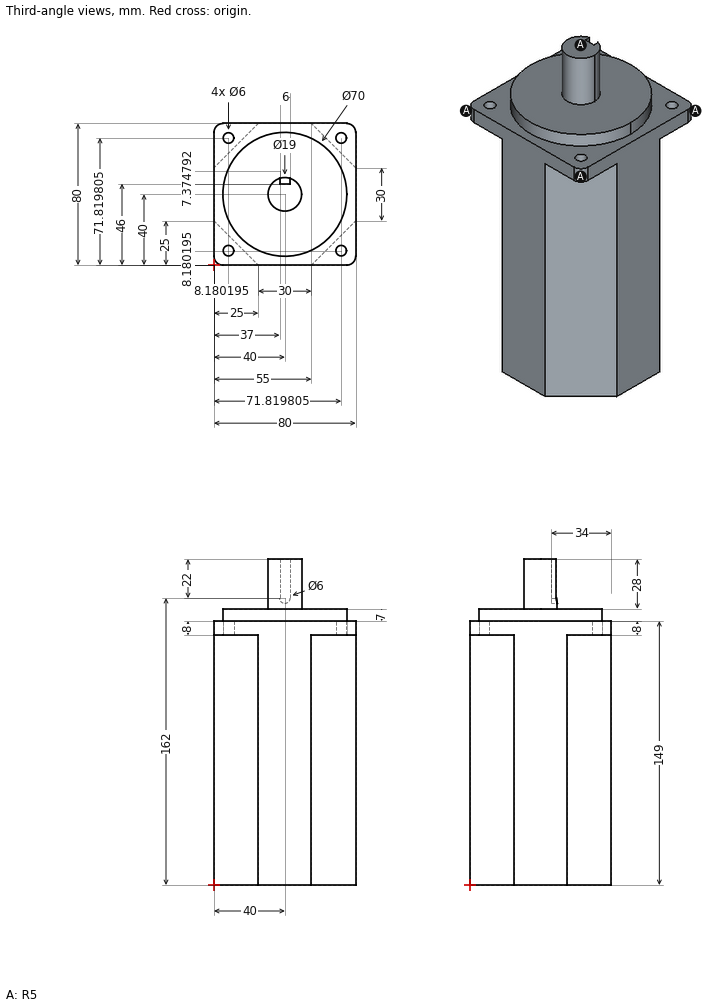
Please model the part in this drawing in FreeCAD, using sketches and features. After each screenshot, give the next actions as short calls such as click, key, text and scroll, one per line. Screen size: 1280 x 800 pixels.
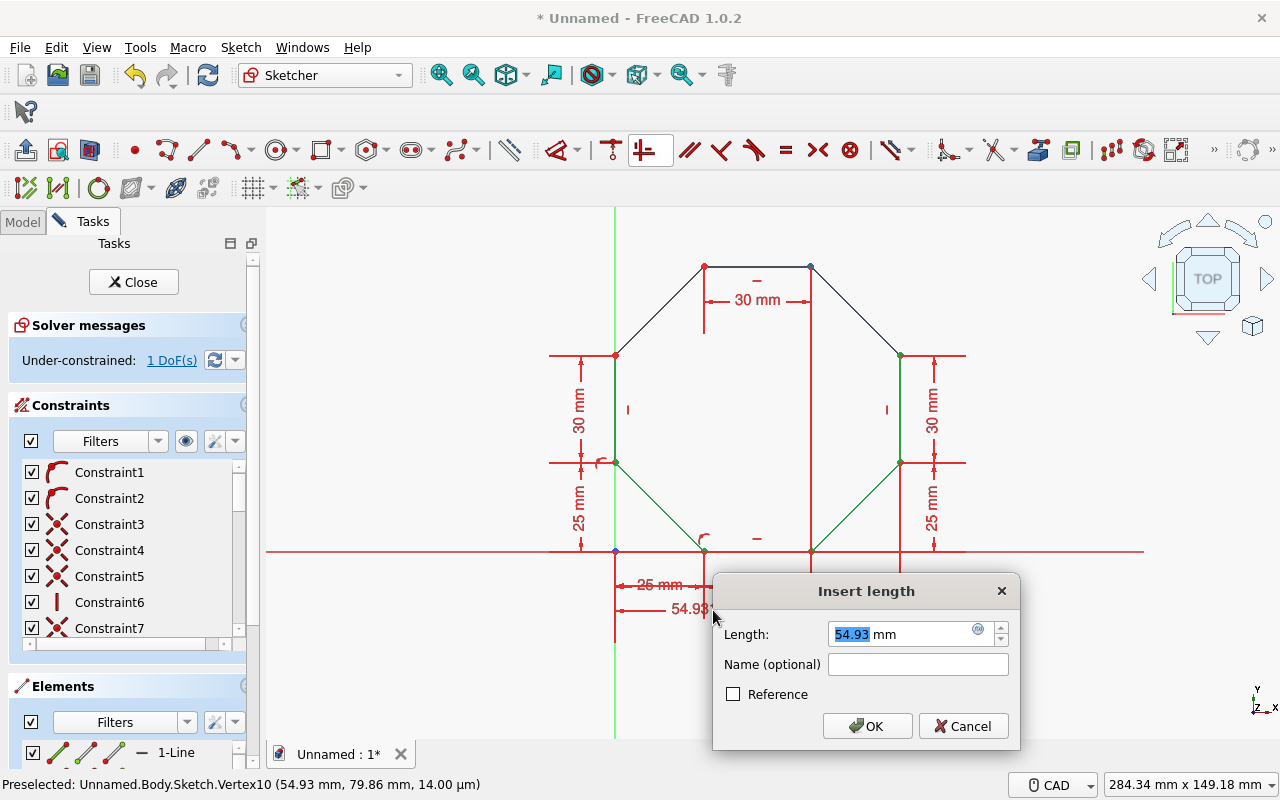
text(55)
key(Return)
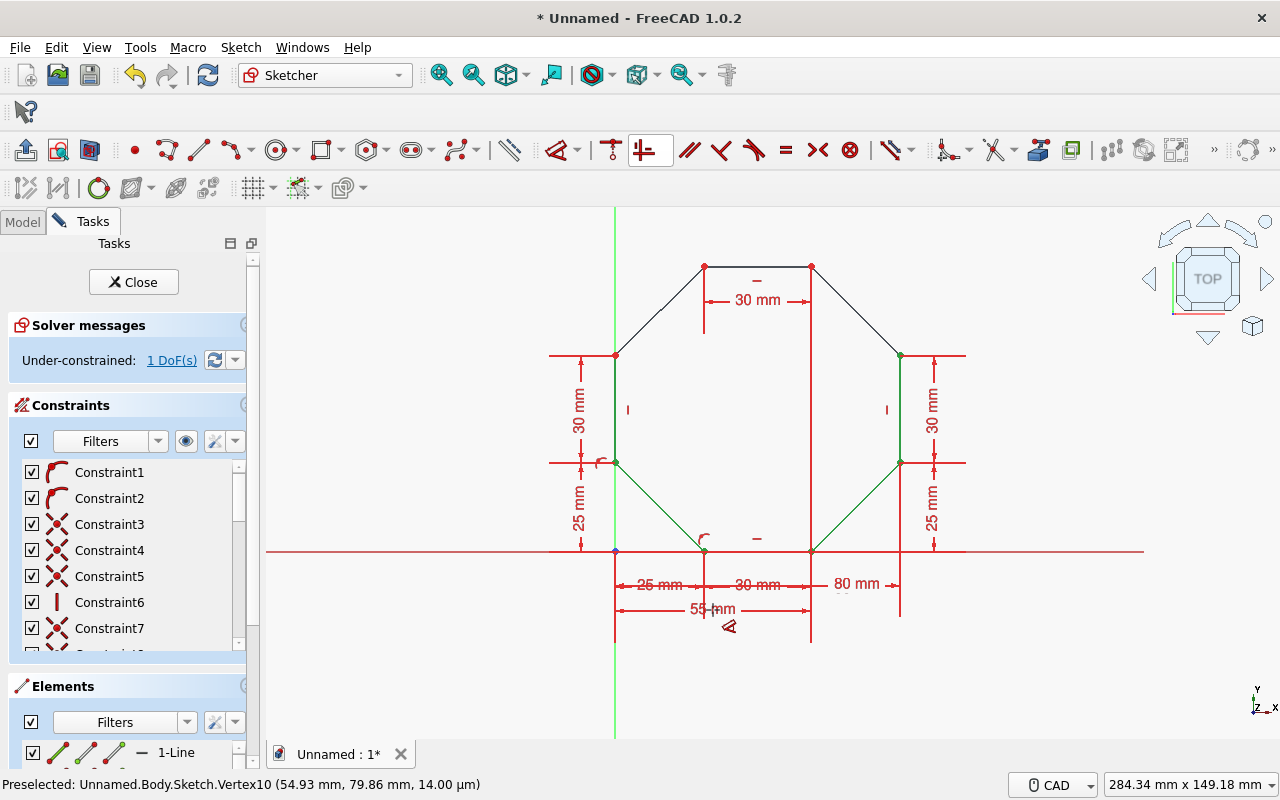
click(811, 267)
click(581, 344)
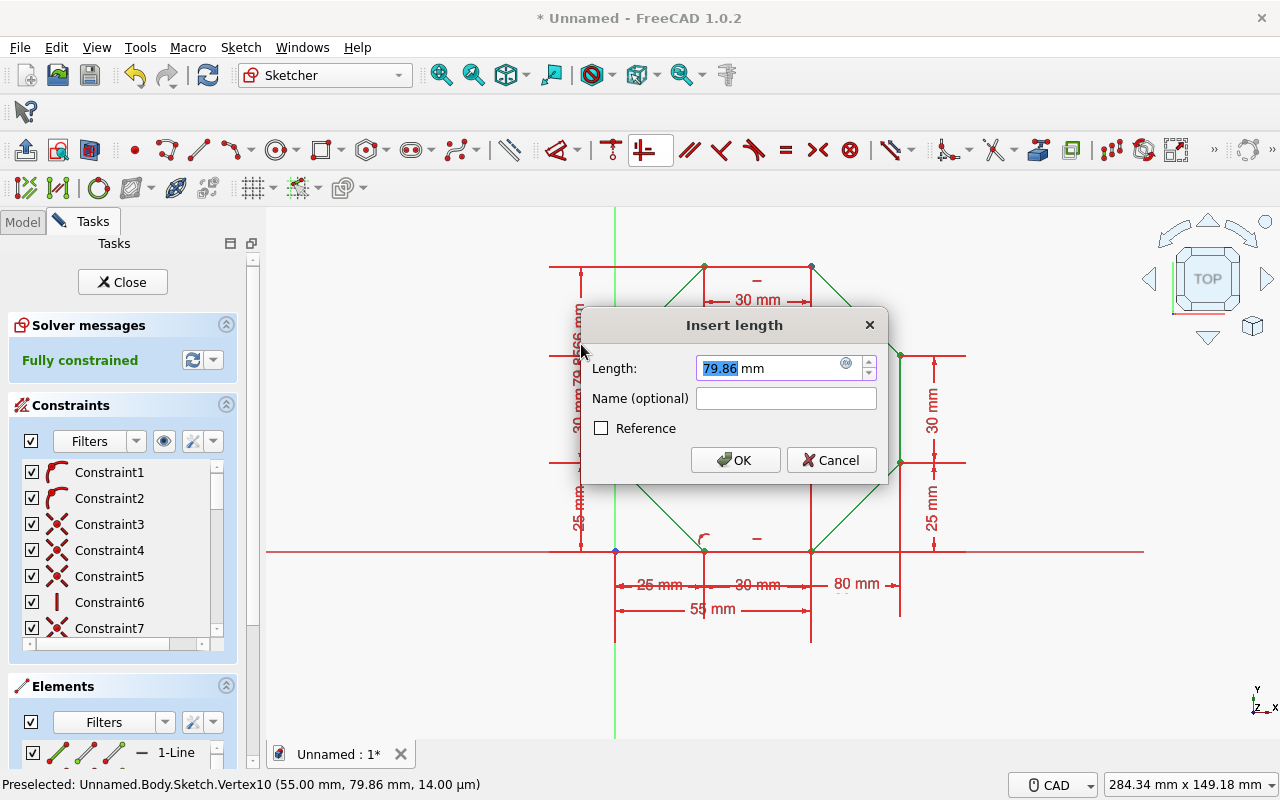
text(80)
key(Return)
key(Escape)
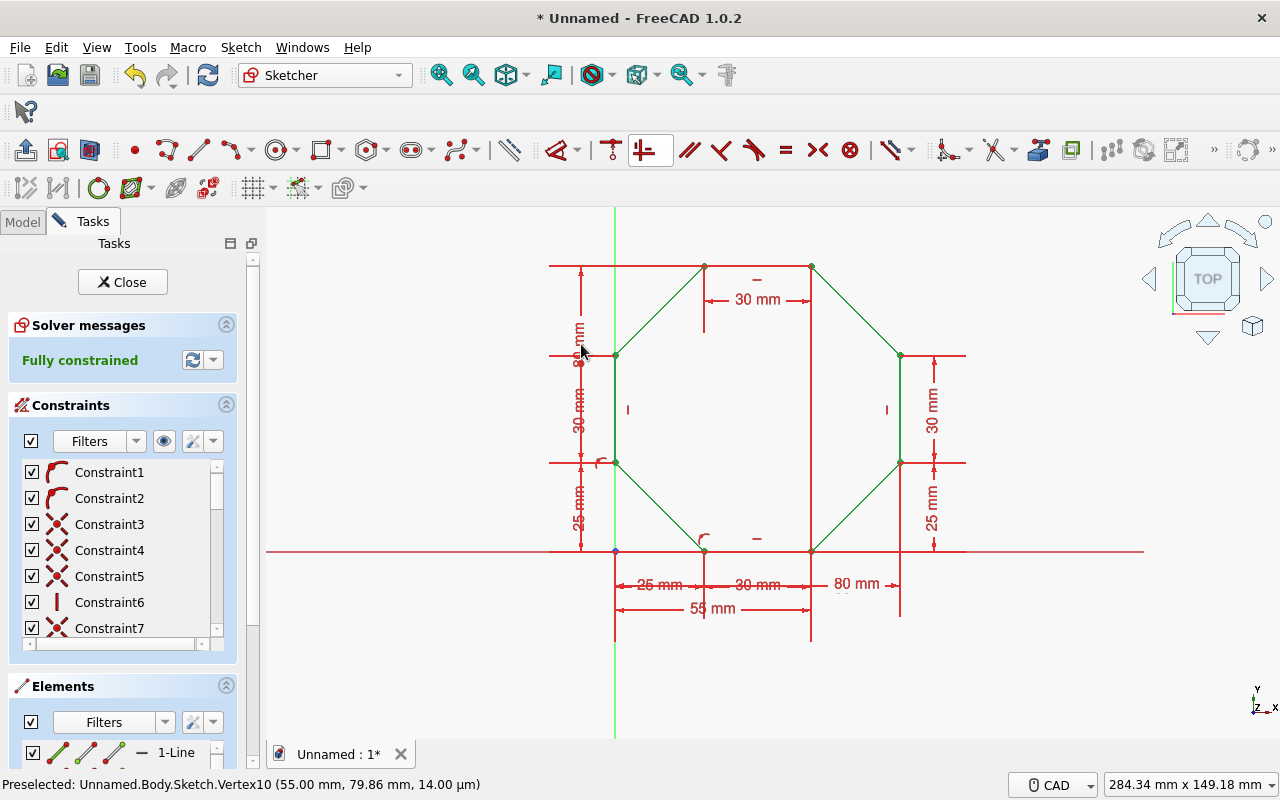
click(123, 282)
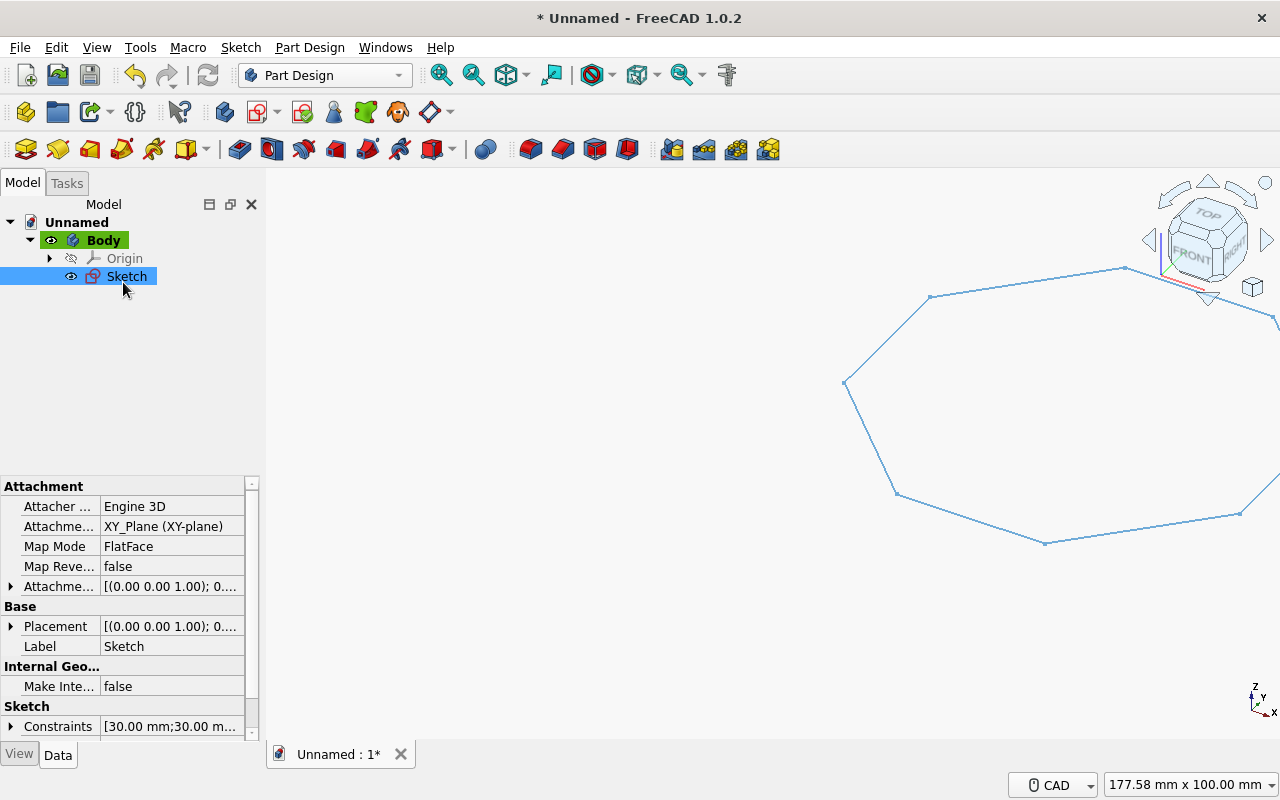
click(26, 150)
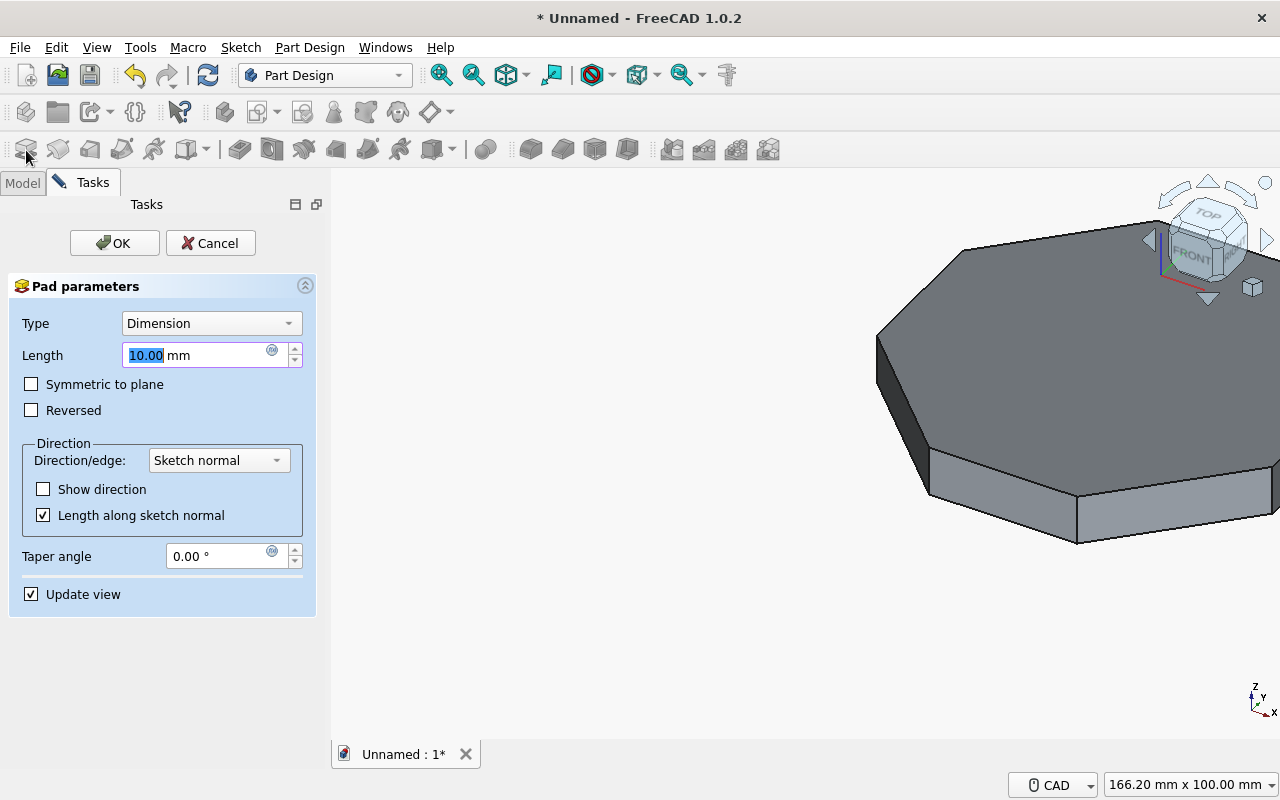
text(149)
key(Tab)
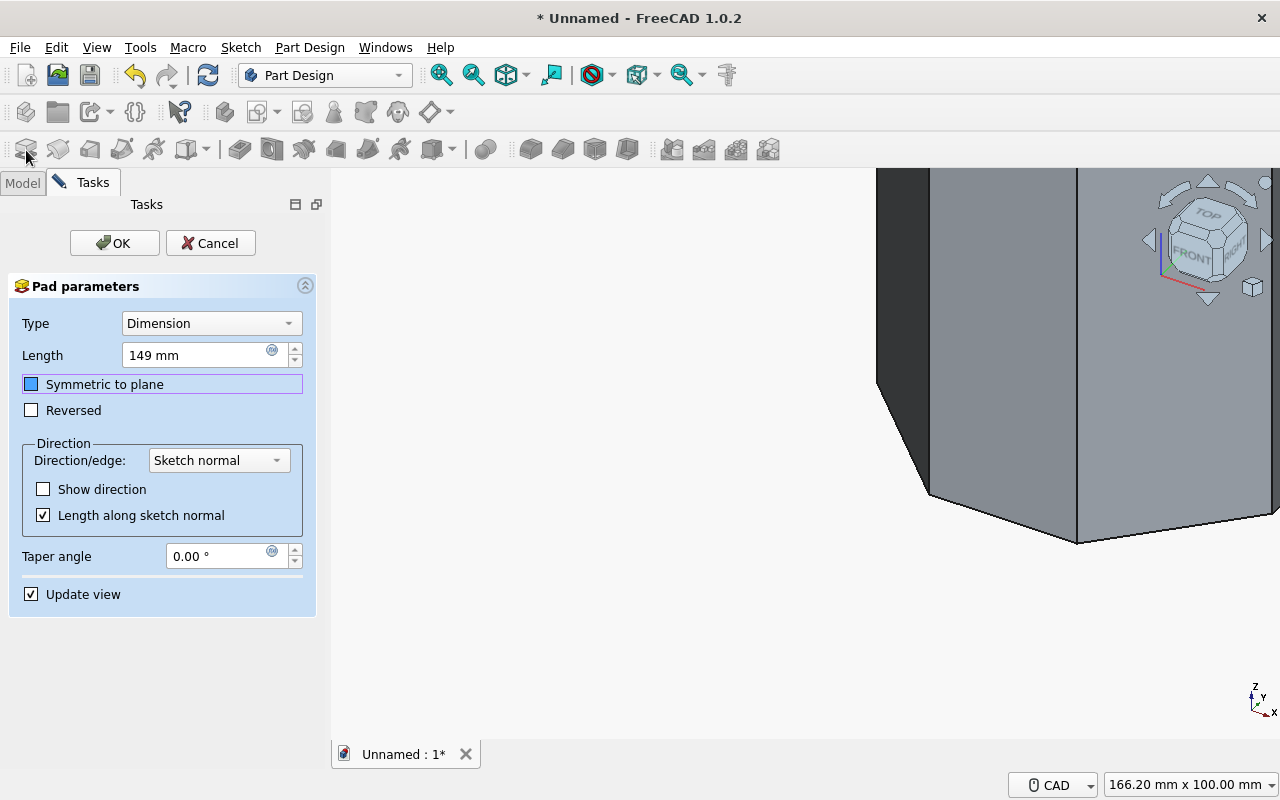
click(115, 243)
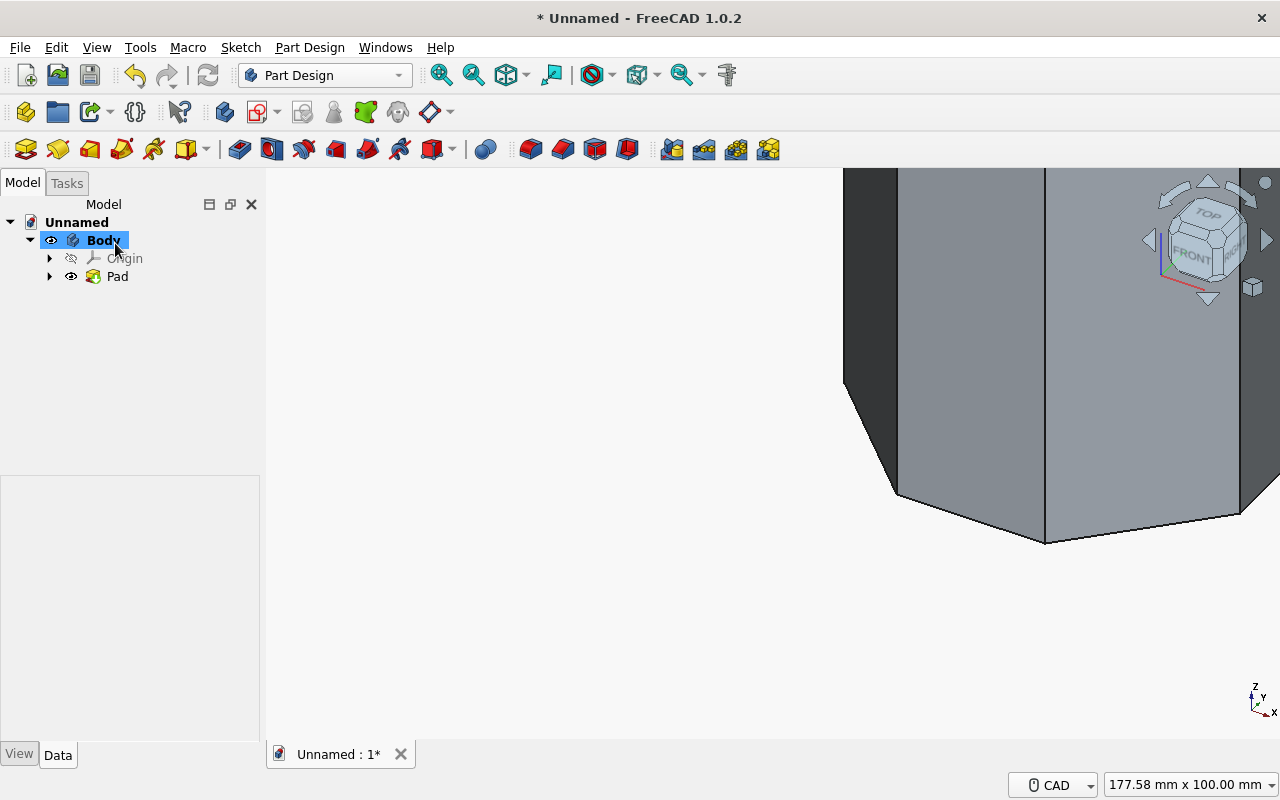
click(442, 76)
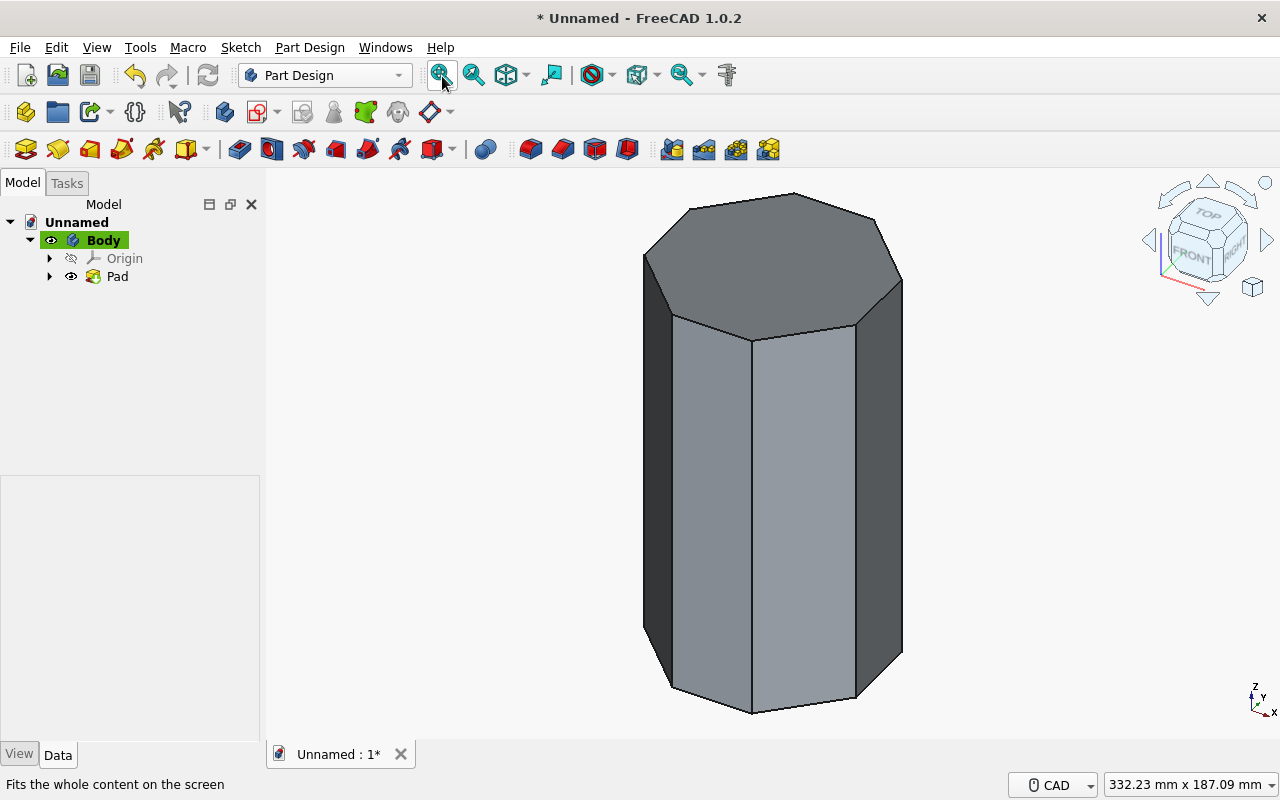
click(773, 266)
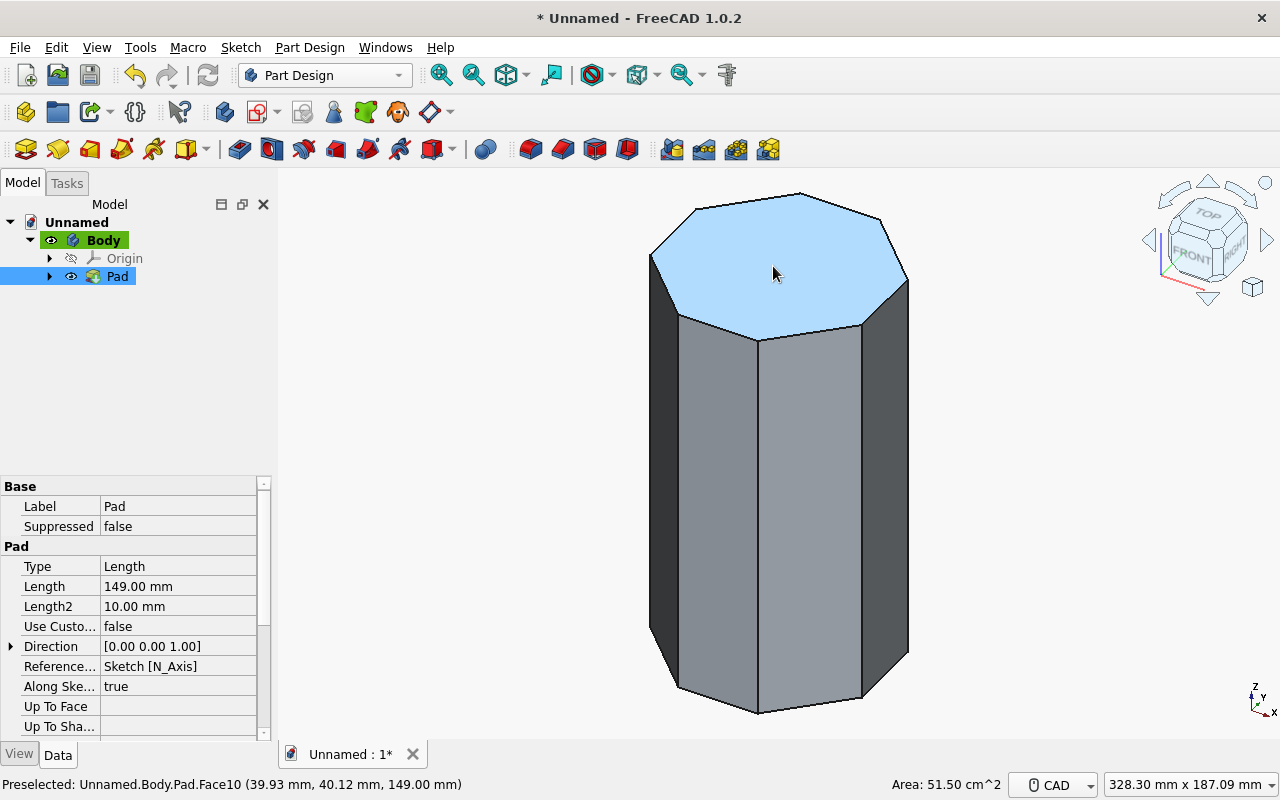
click(258, 112)